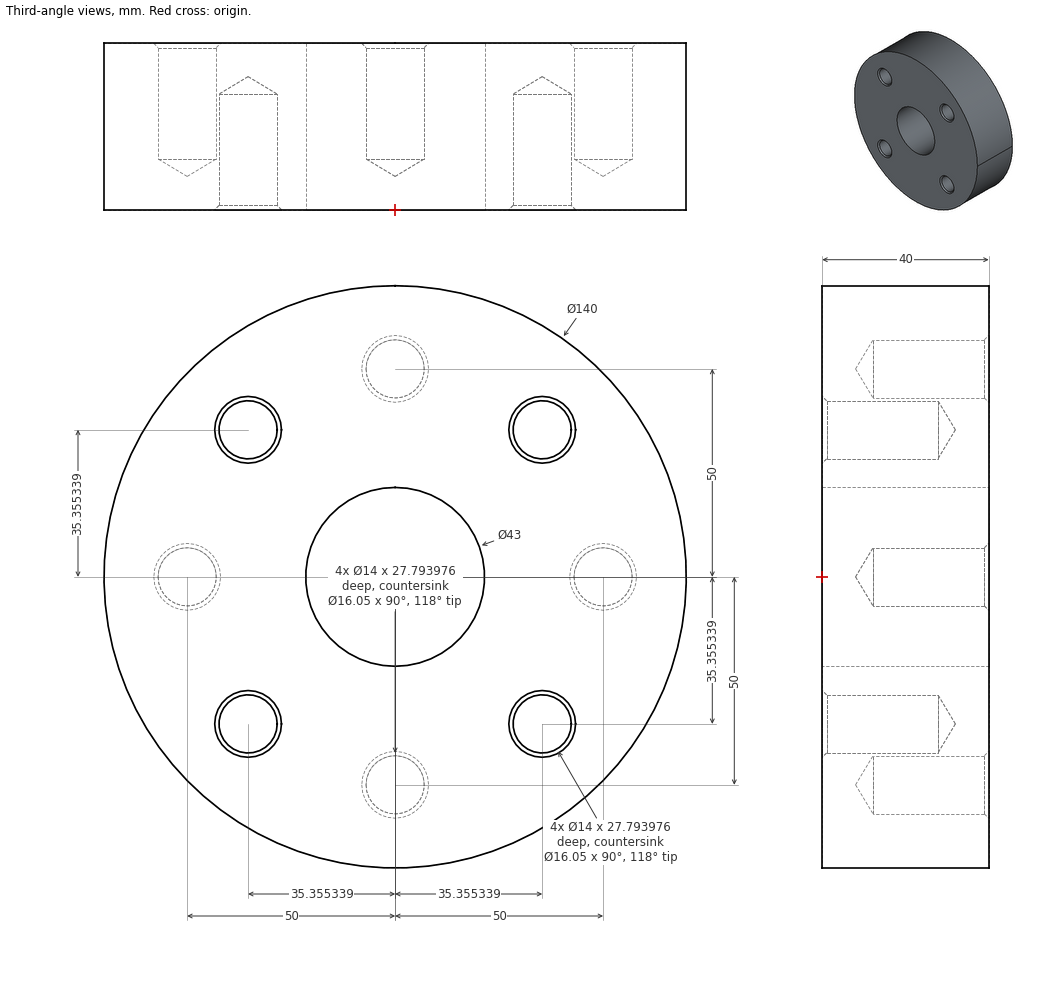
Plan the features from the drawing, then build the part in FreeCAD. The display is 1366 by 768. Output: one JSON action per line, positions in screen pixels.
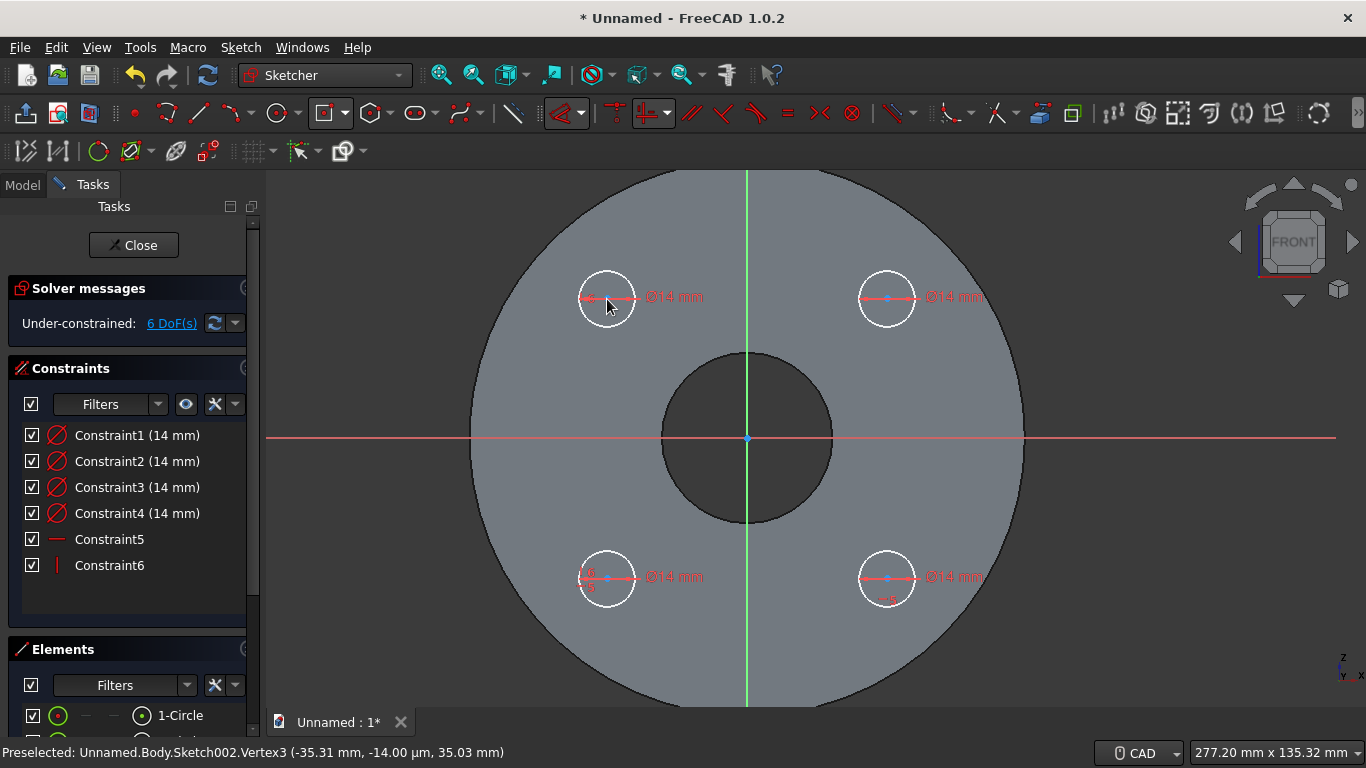
{"action": "left_click", "coordinate": [887, 579]}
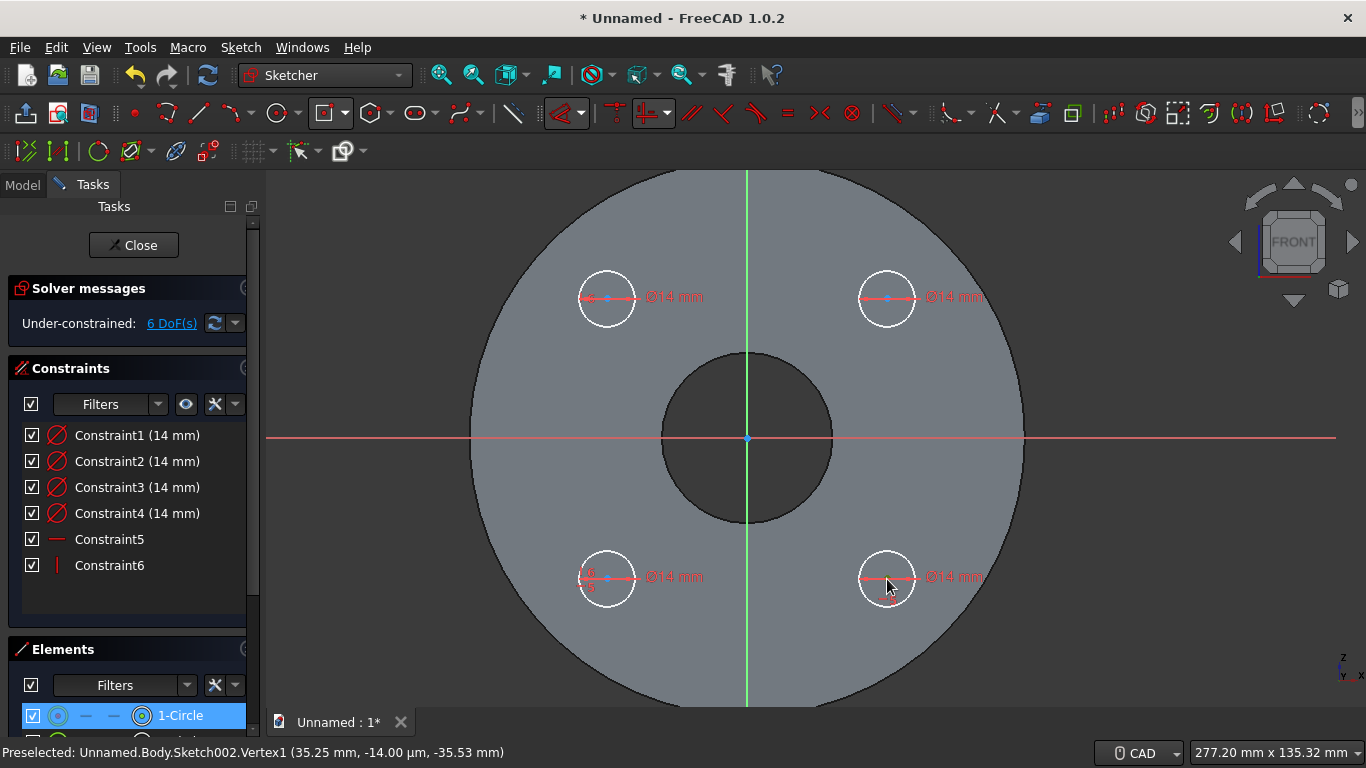
{"action": "left_click", "coordinate": [887, 299]}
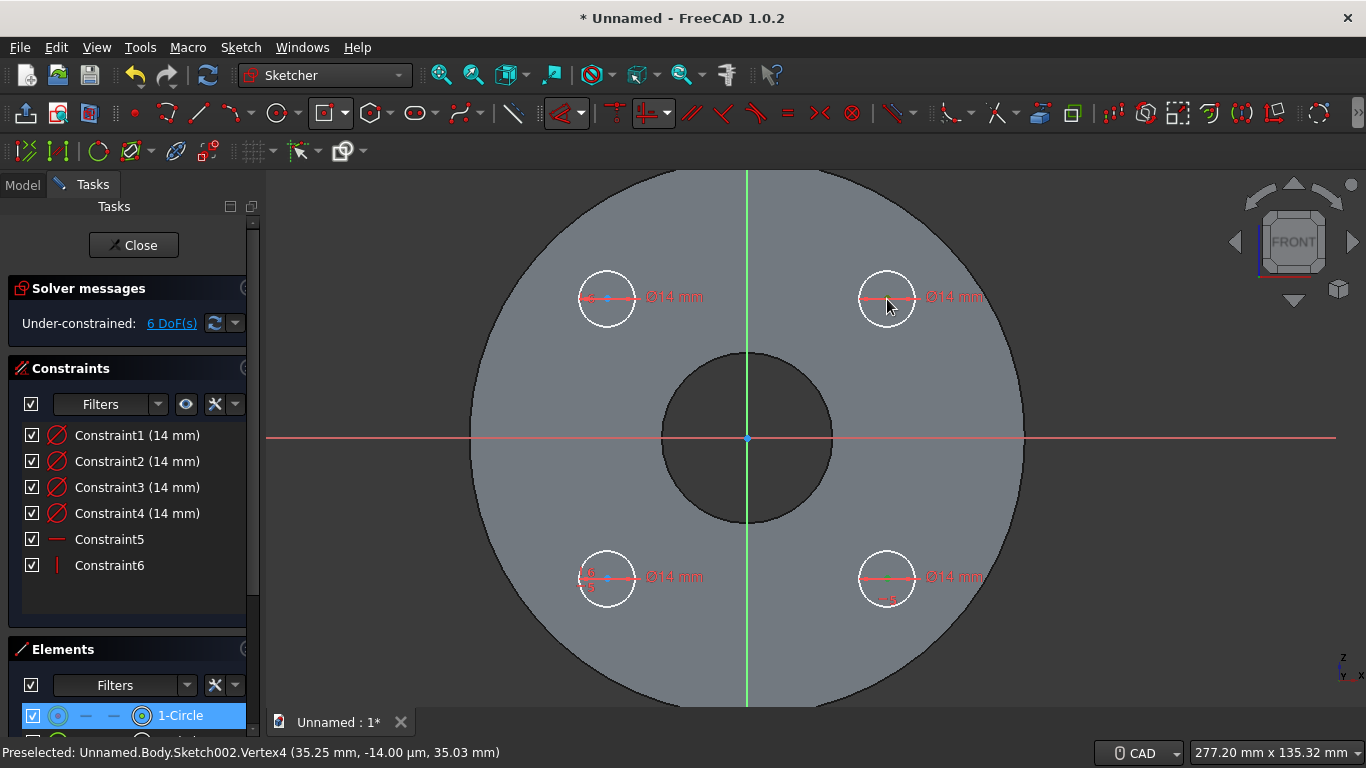
{"action": "left_click", "coordinate": [670, 114]}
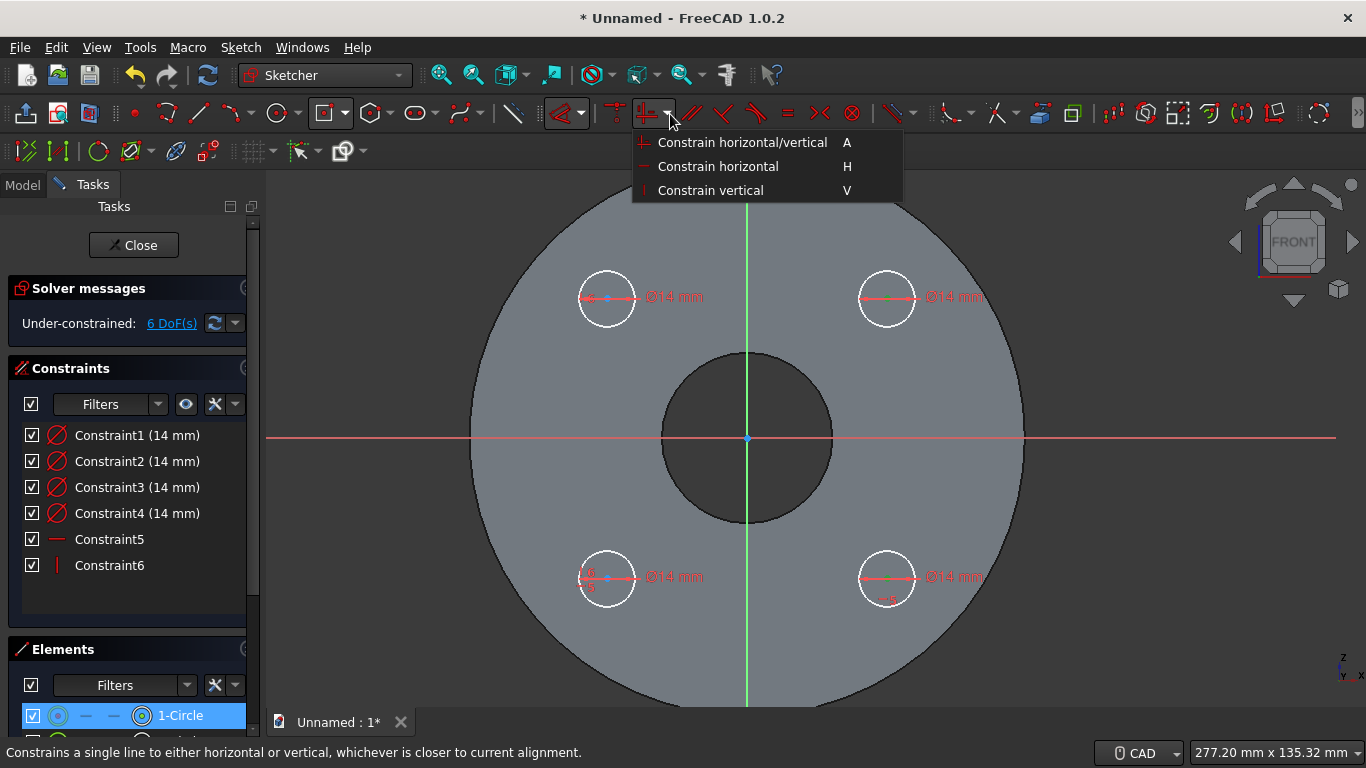
{"action": "left_click", "coordinate": [768, 190]}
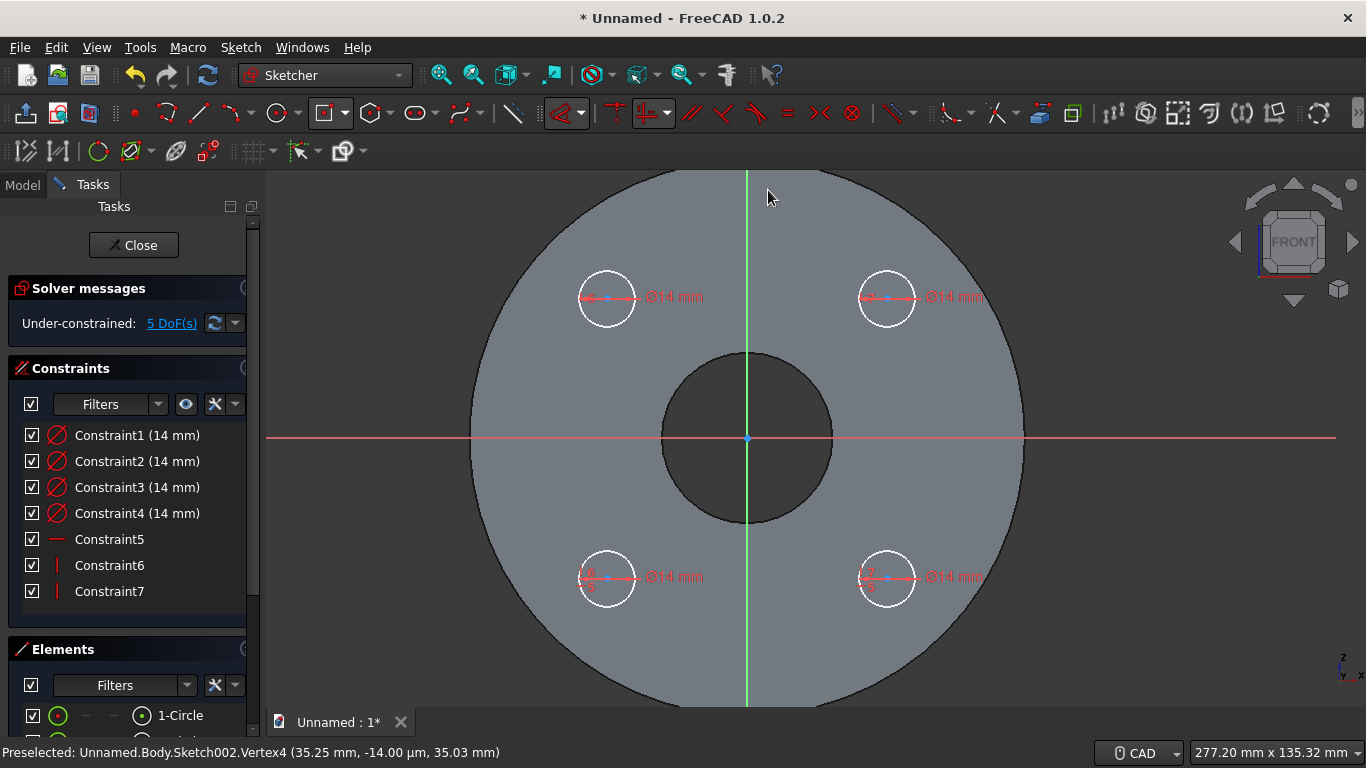
{"action": "left_click", "coordinate": [607, 299]}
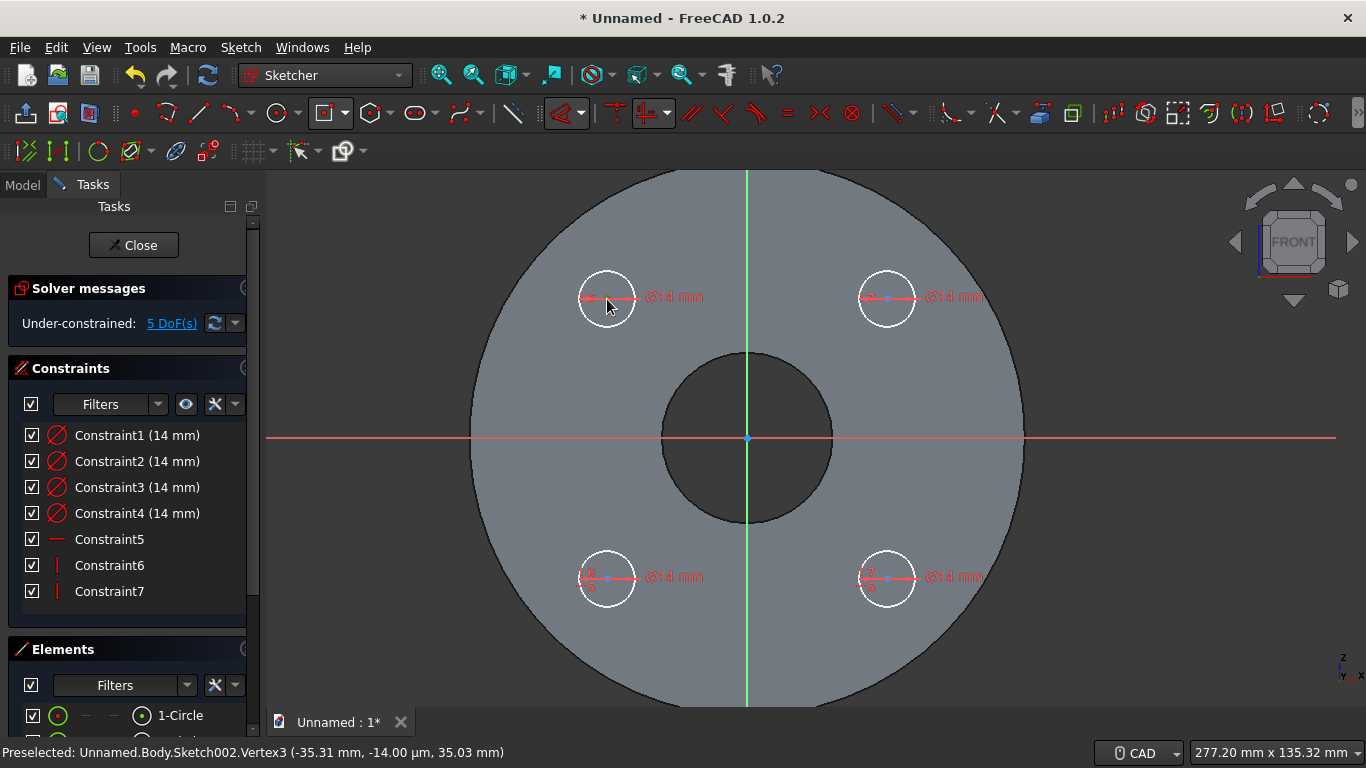
{"action": "left_click", "coordinate": [887, 299]}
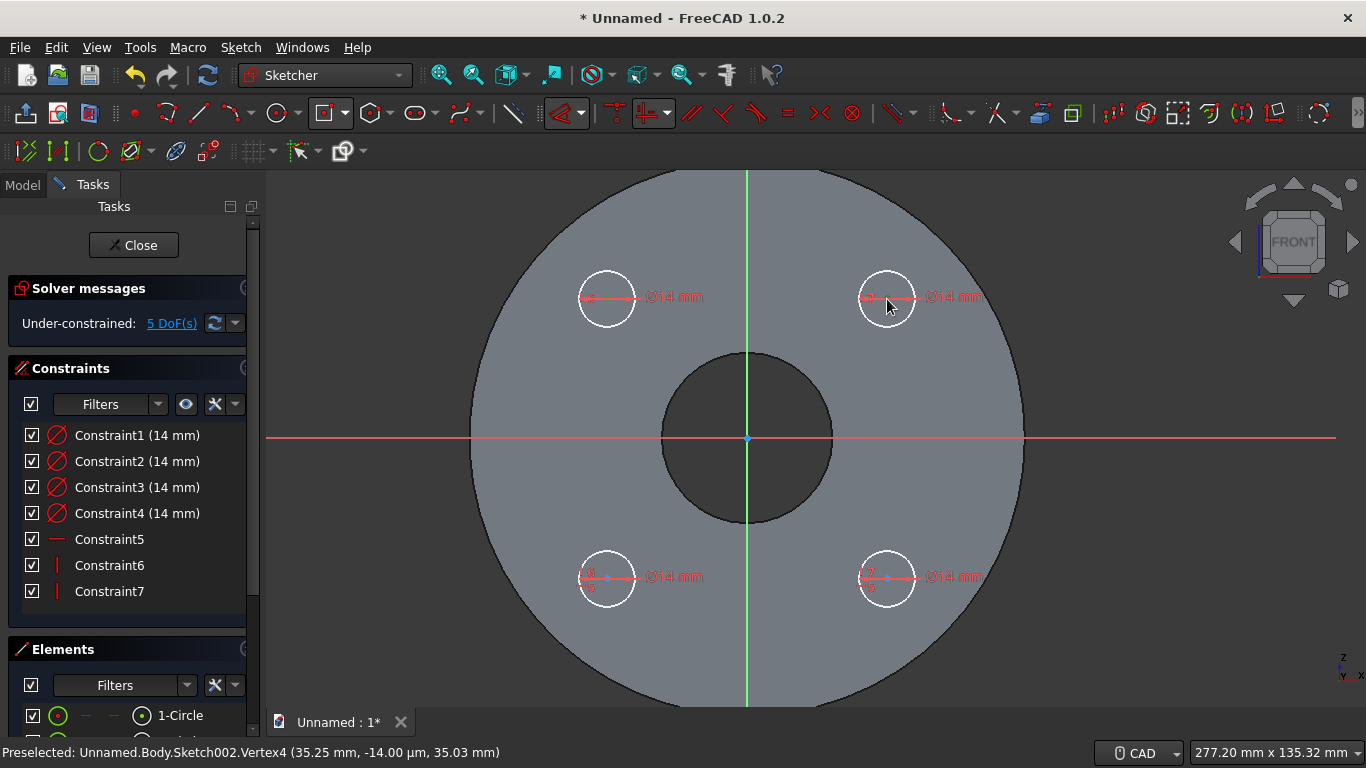
{"action": "key", "text": "h"}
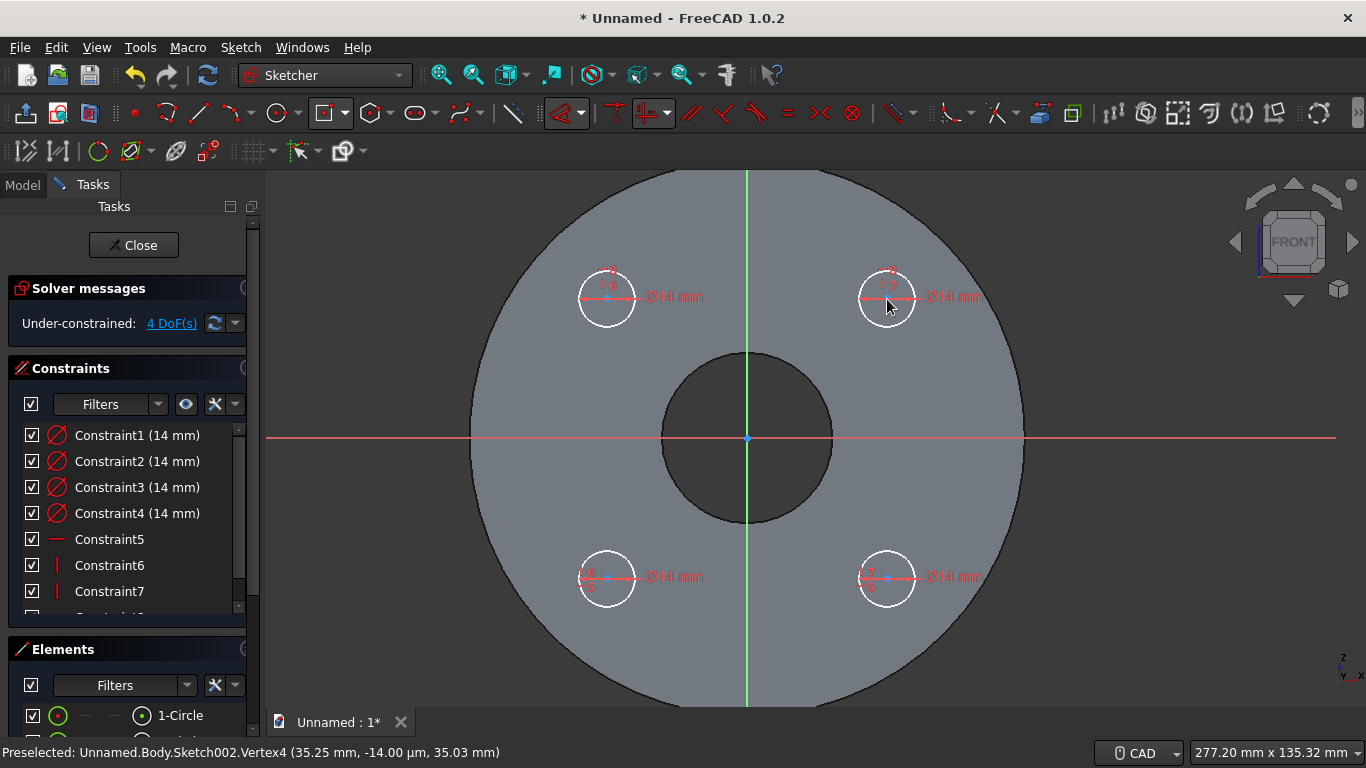
{"action": "left_click", "coordinate": [887, 579]}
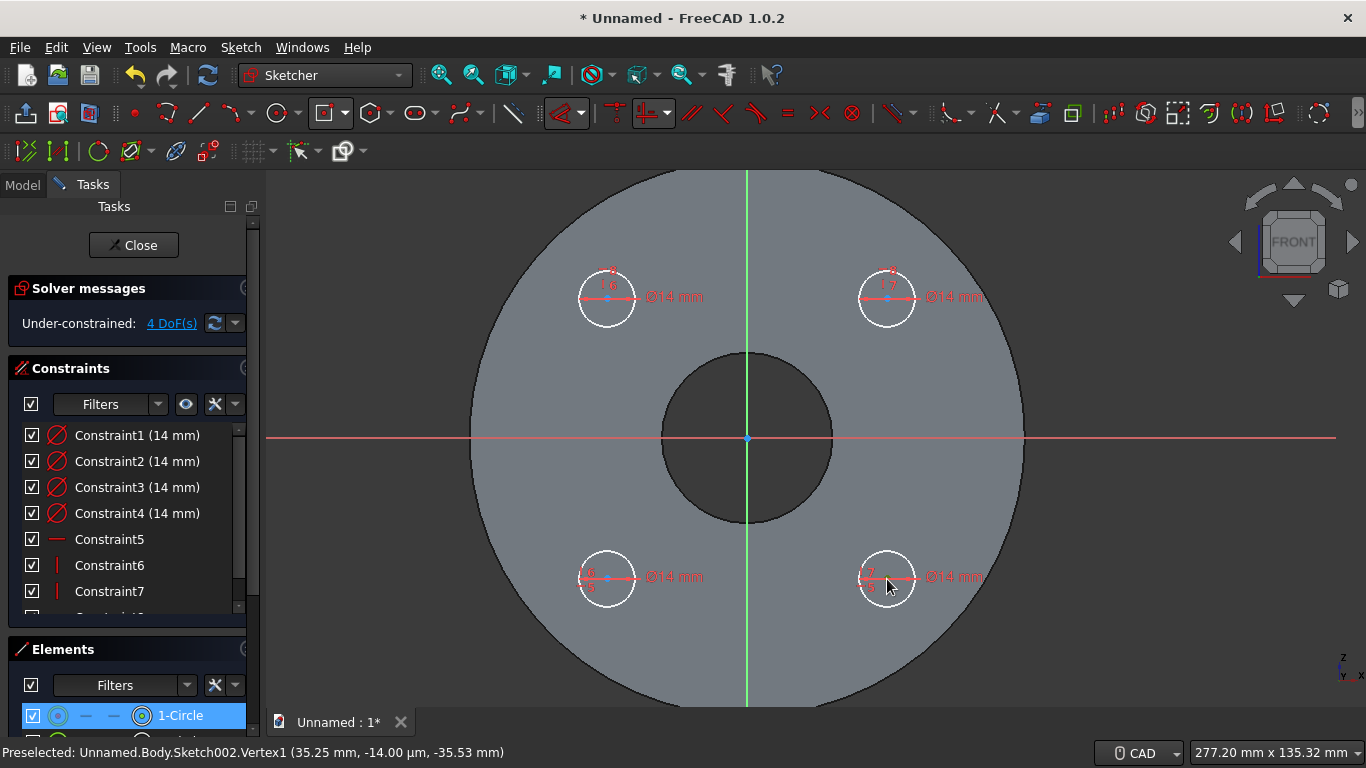
{"action": "left_click", "coordinate": [584, 114]}